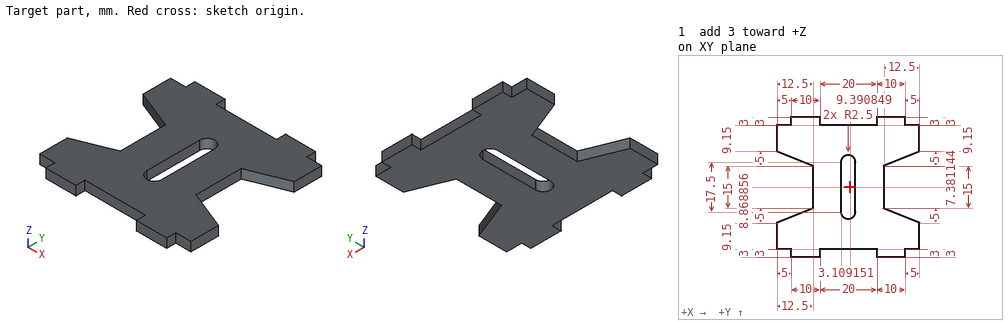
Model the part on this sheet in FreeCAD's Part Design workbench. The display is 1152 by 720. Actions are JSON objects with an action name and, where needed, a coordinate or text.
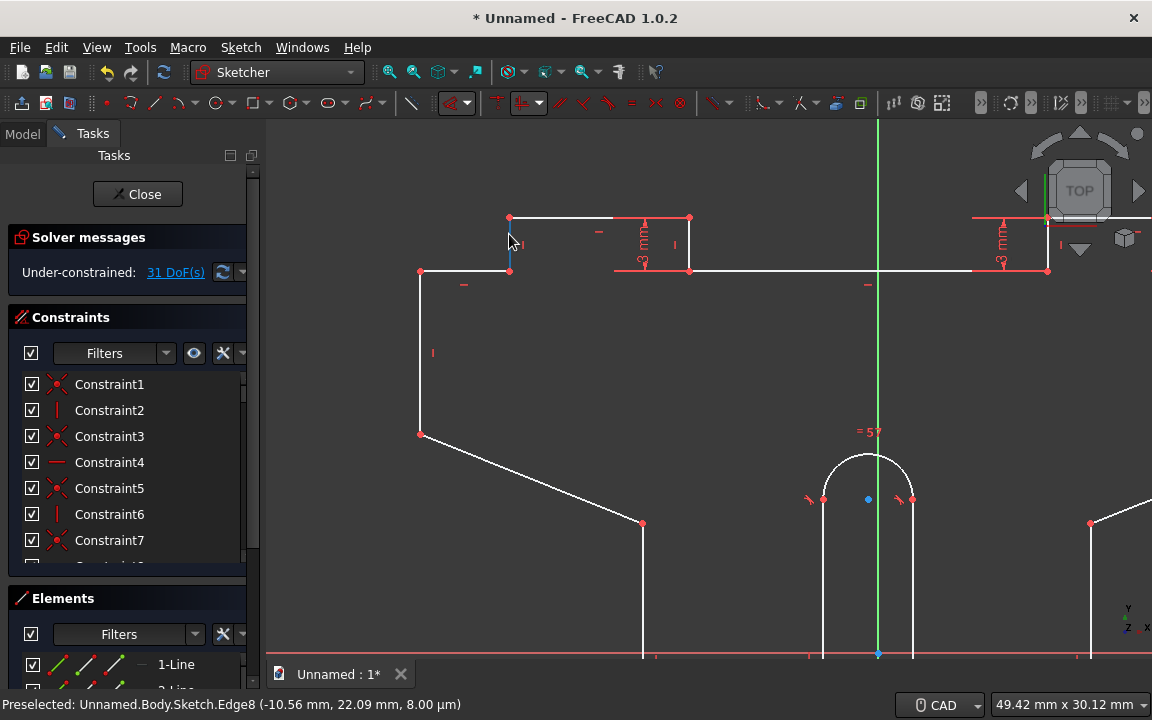
{"action": "left_click", "coordinate": [510, 234]}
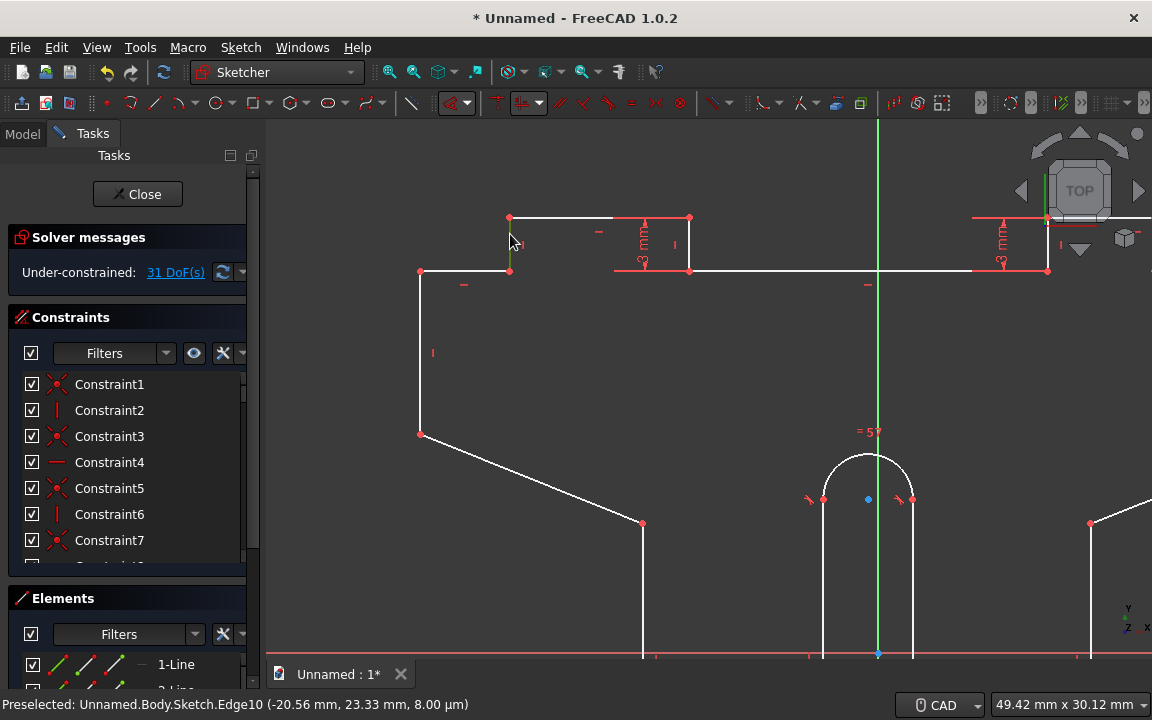
{"action": "left_click", "coordinate": [470, 104]}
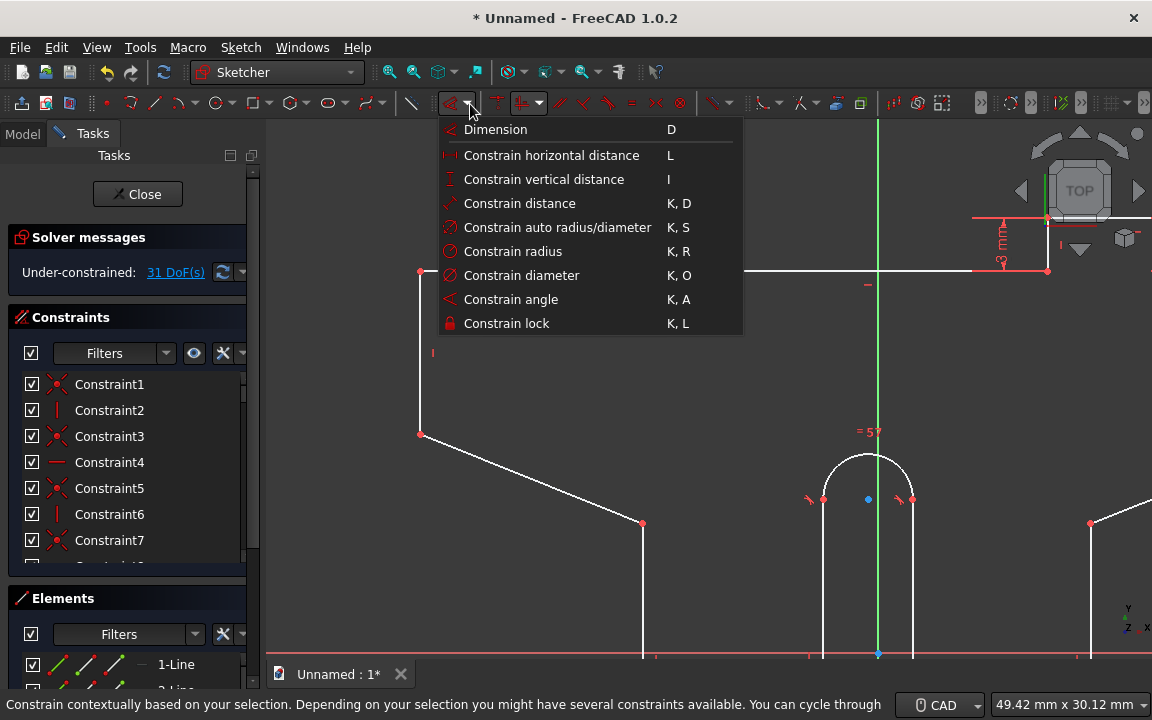
{"action": "left_click", "coordinate": [591, 179]}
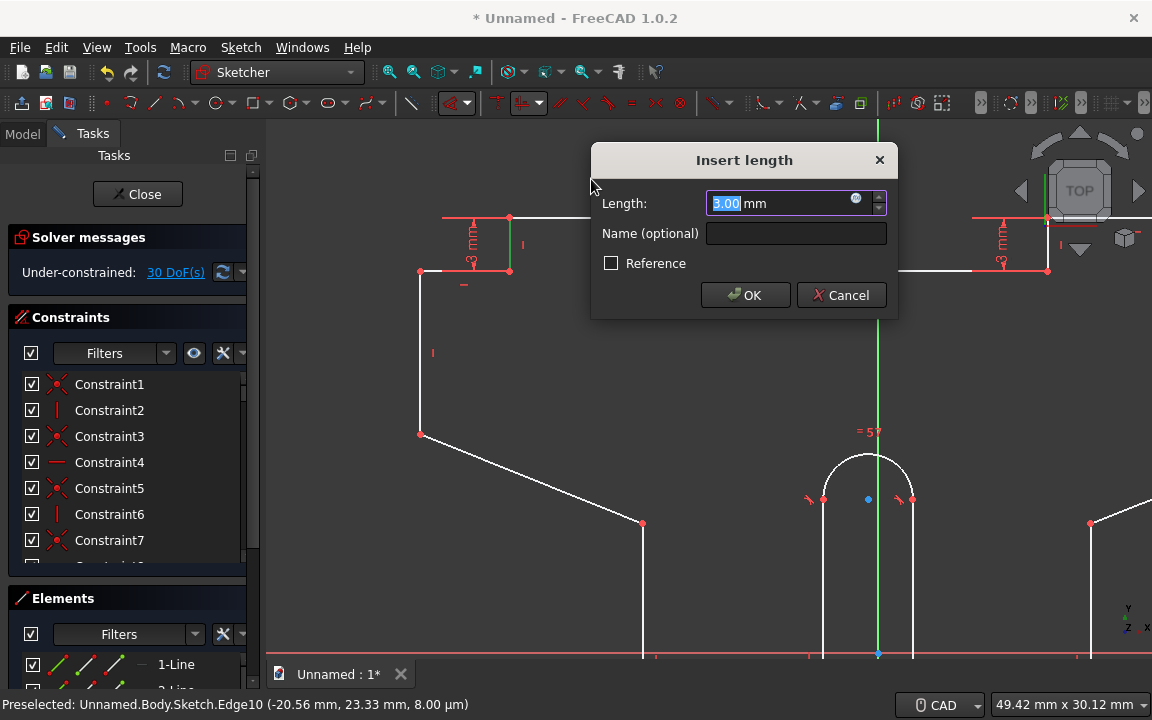
{"action": "type", "text": "3"}
{"action": "key", "text": "Return"}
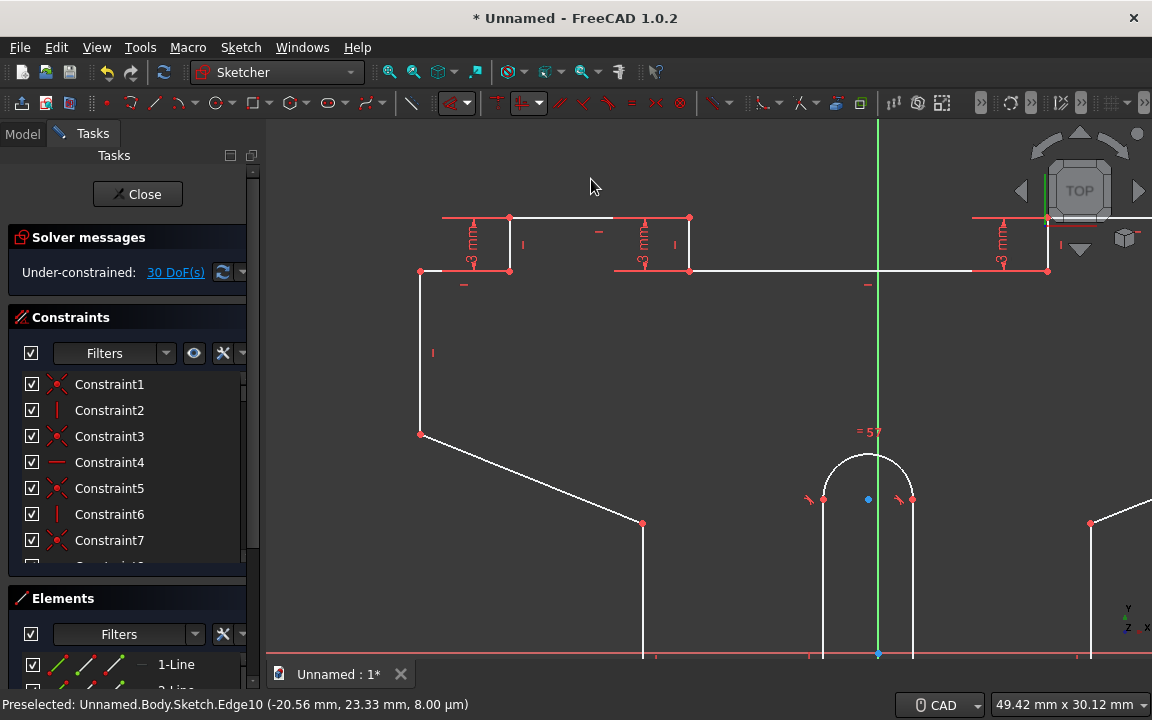
{"action": "left_click", "coordinate": [483, 271]}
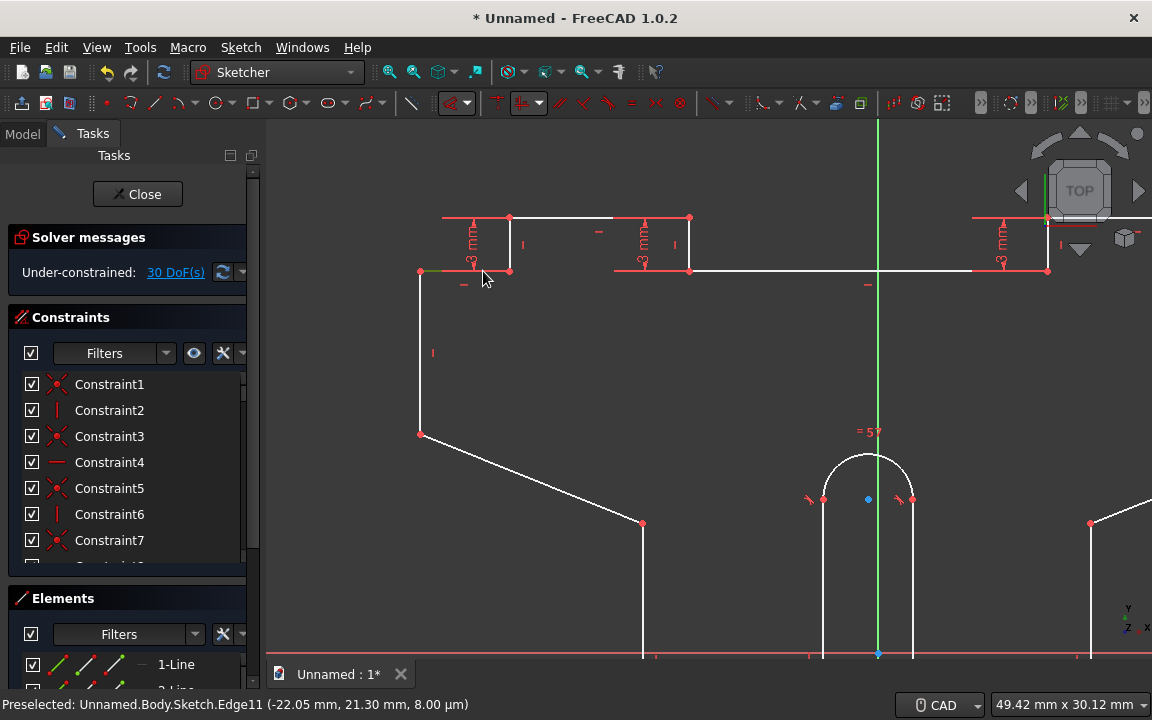
{"action": "left_click", "coordinate": [470, 104]}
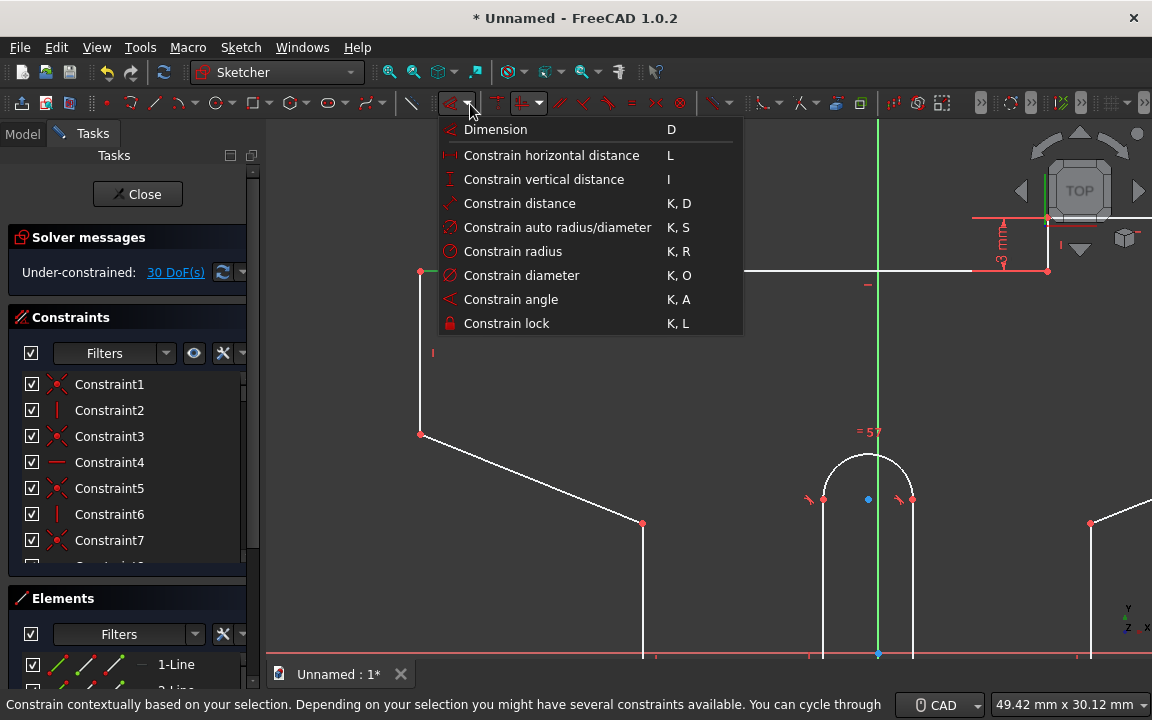
{"action": "left_click", "coordinate": [591, 155]}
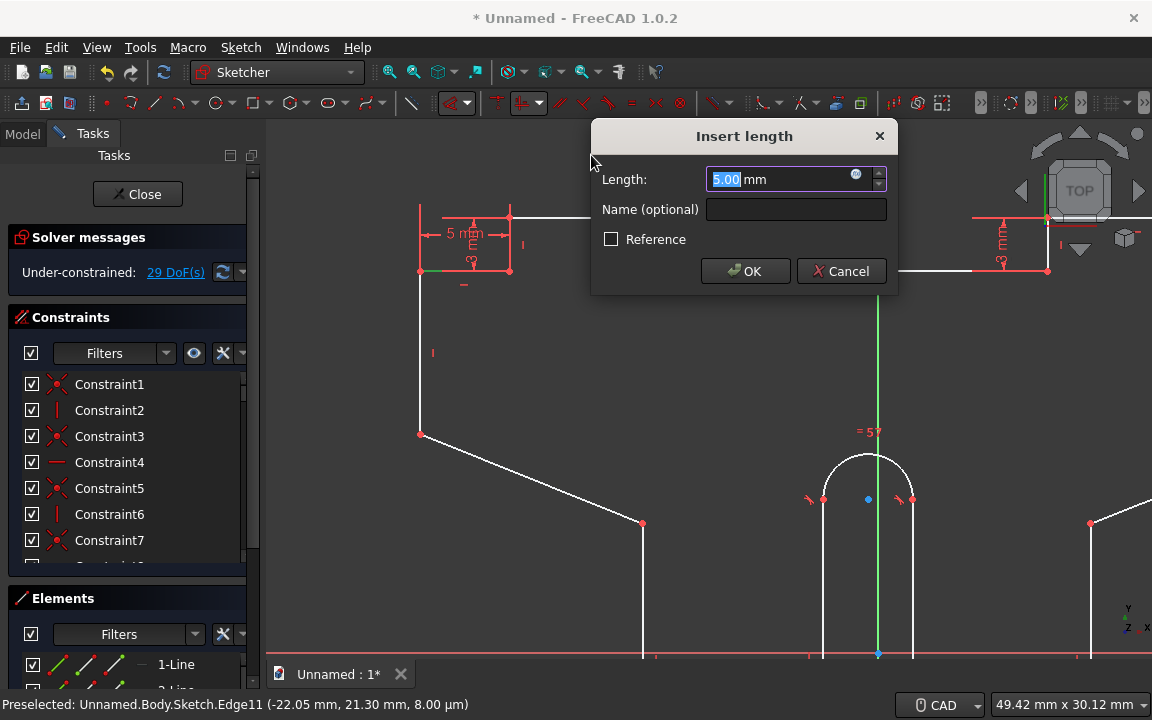
{"action": "type", "text": "5"}
{"action": "key", "text": "Return"}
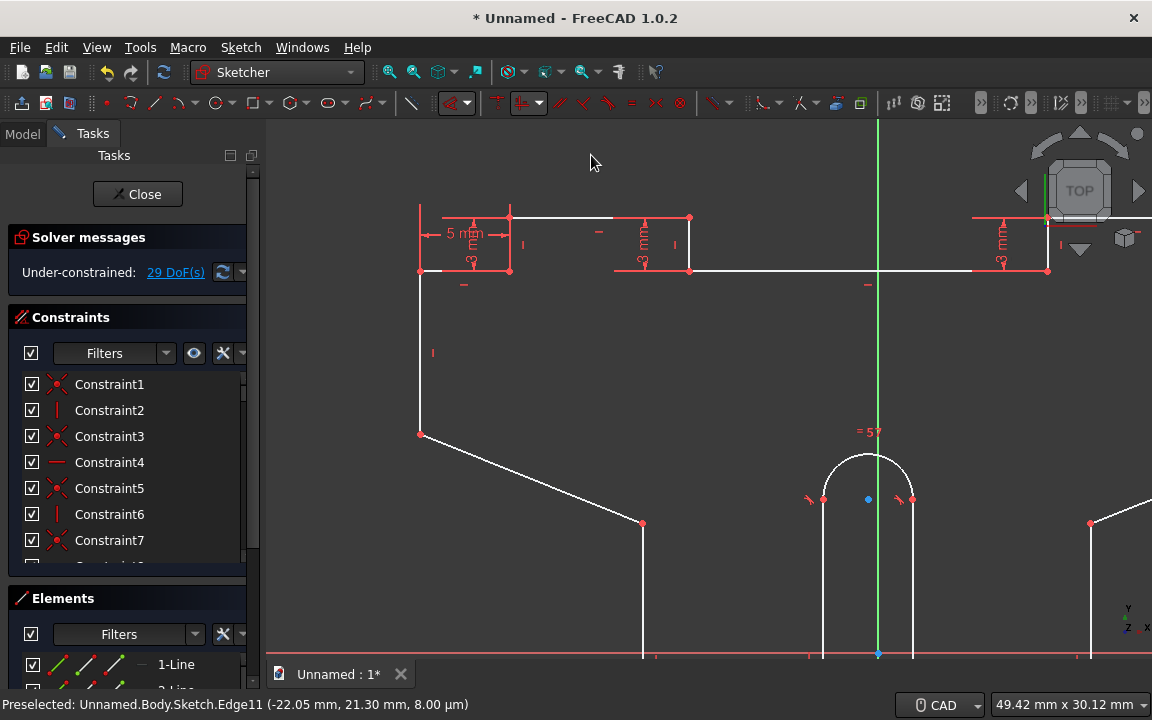
{"action": "scroll", "coordinate": [508, 234], "scroll_direction": "down", "scroll_amount": 5}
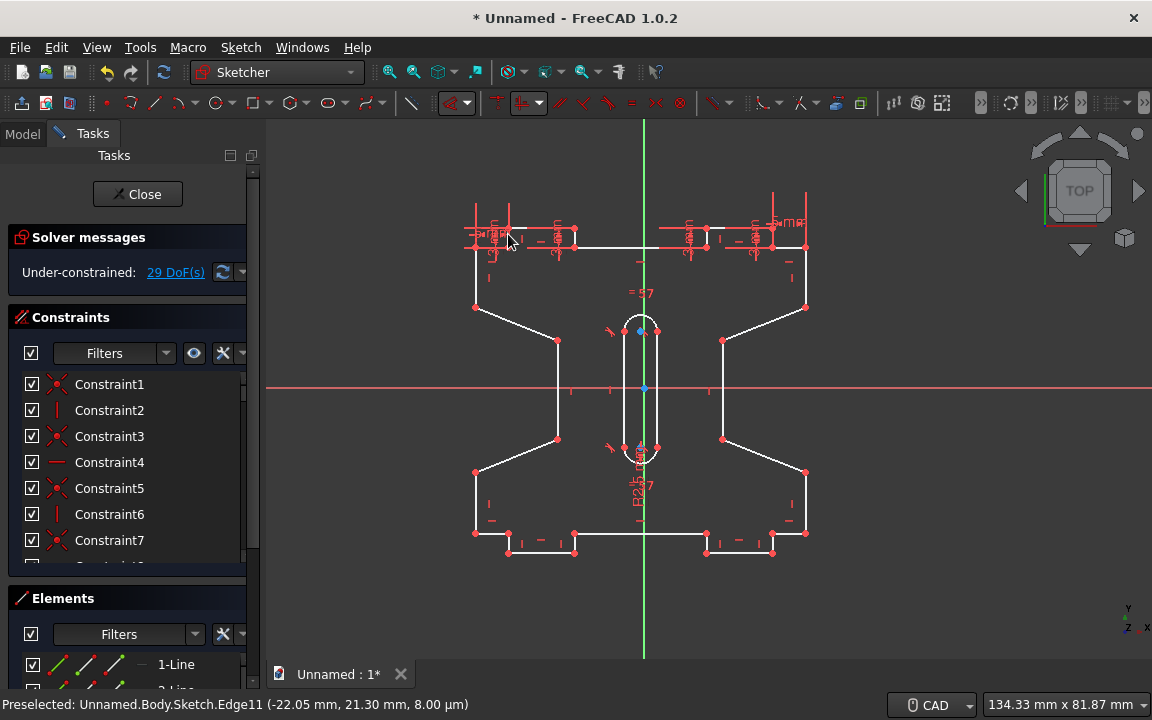
{"action": "scroll", "coordinate": [486, 534], "scroll_direction": "up", "scroll_amount": 2}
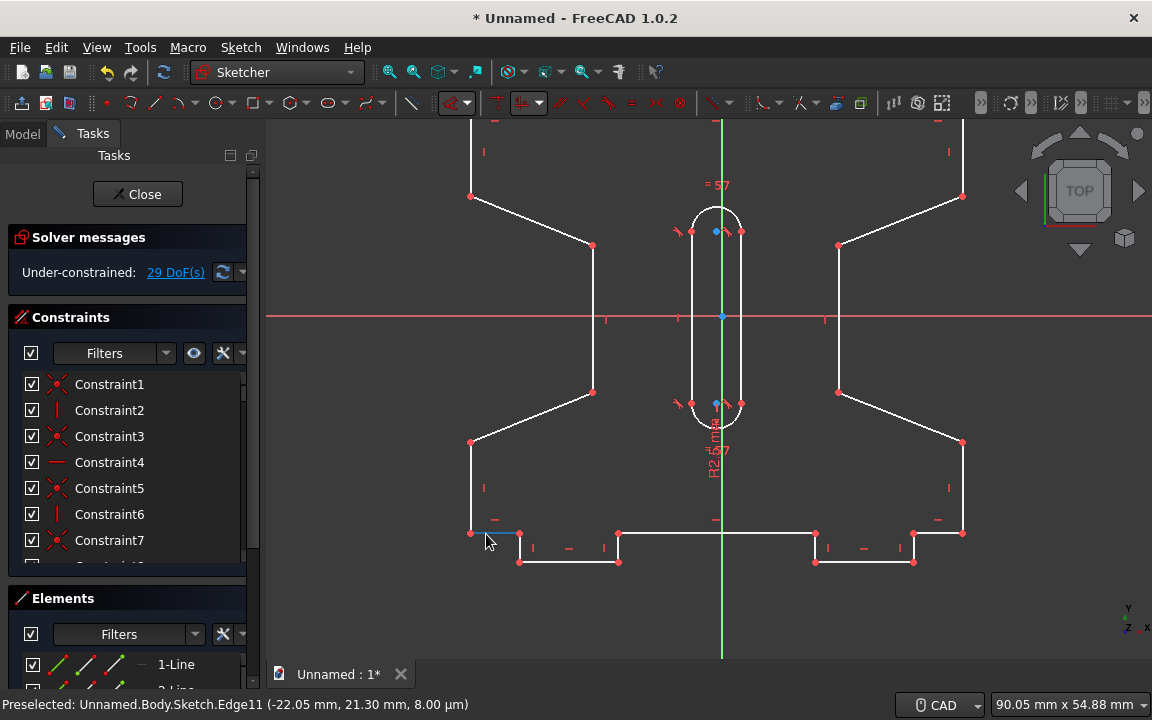
{"action": "left_click", "coordinate": [486, 533]}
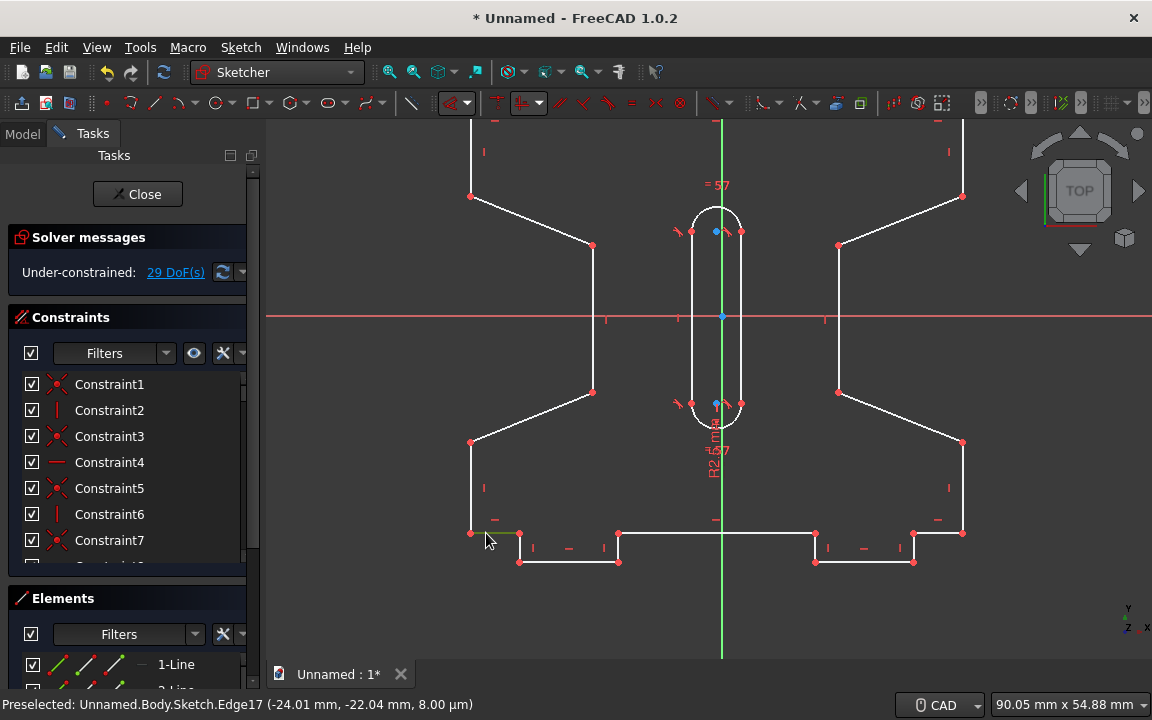
{"action": "left_click", "coordinate": [470, 104]}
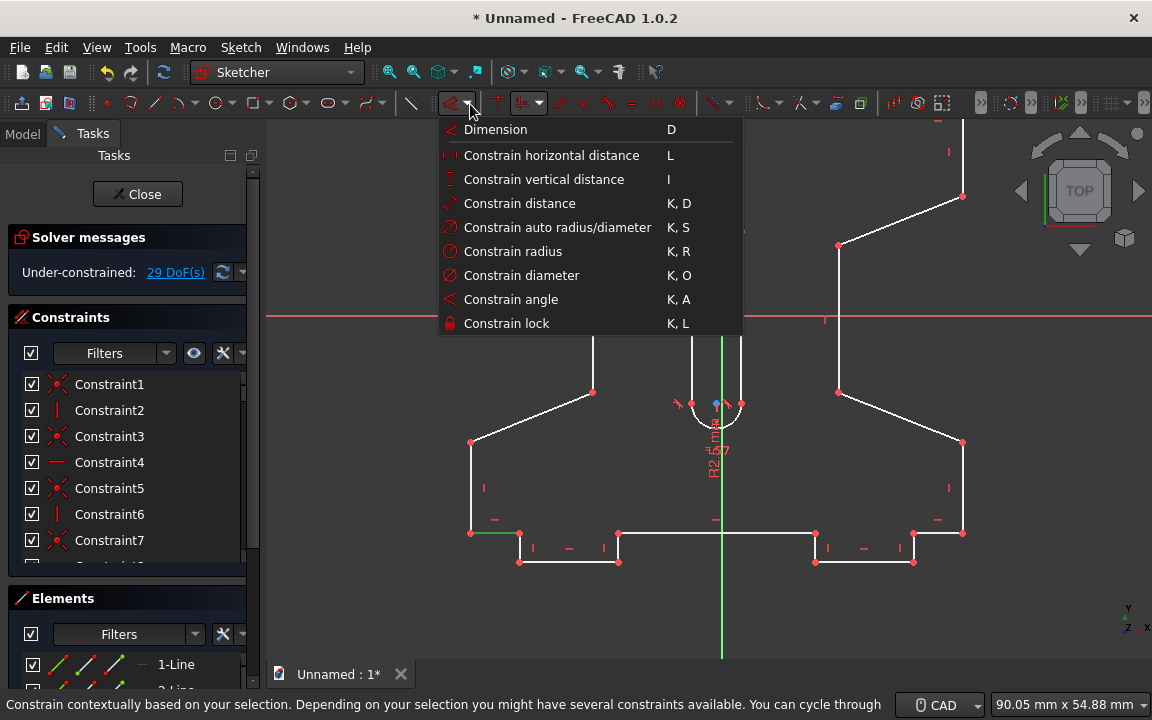
{"action": "left_click", "coordinate": [591, 155]}